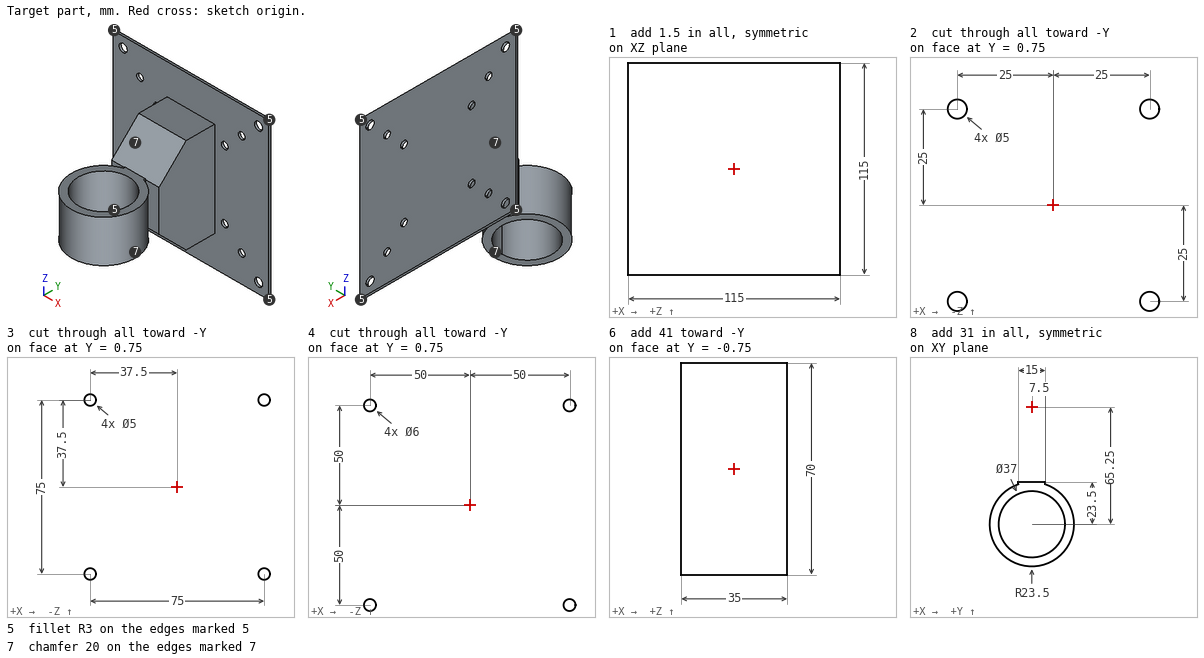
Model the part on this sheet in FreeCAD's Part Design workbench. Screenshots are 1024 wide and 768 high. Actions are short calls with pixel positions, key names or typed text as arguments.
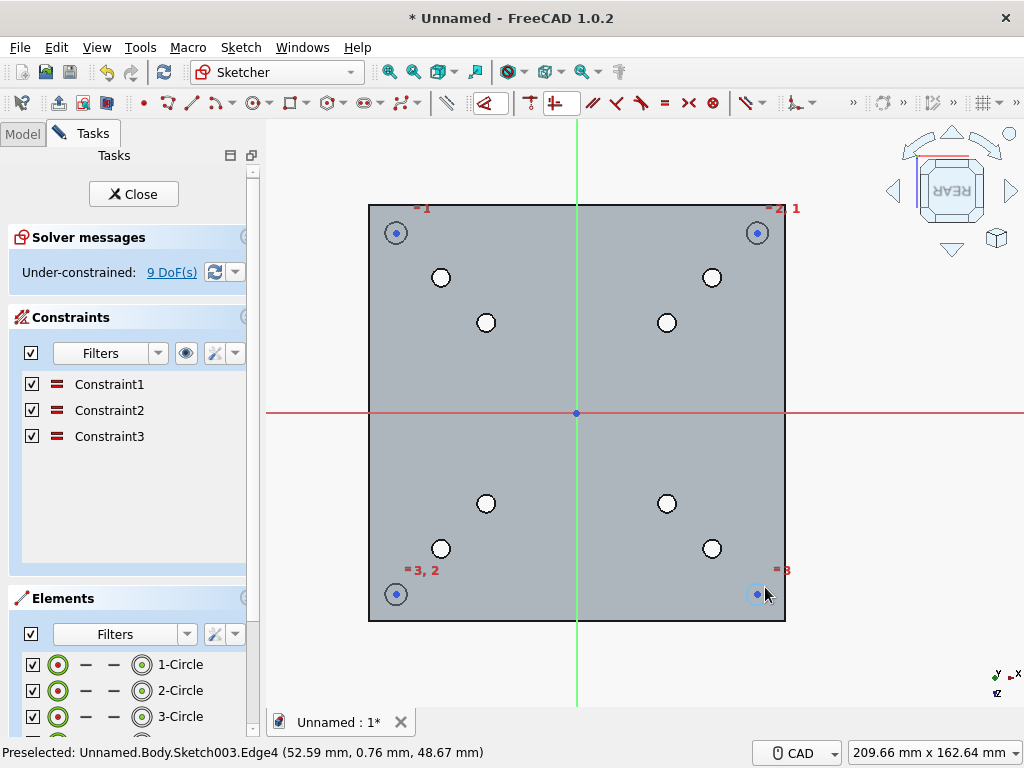
click(396, 233)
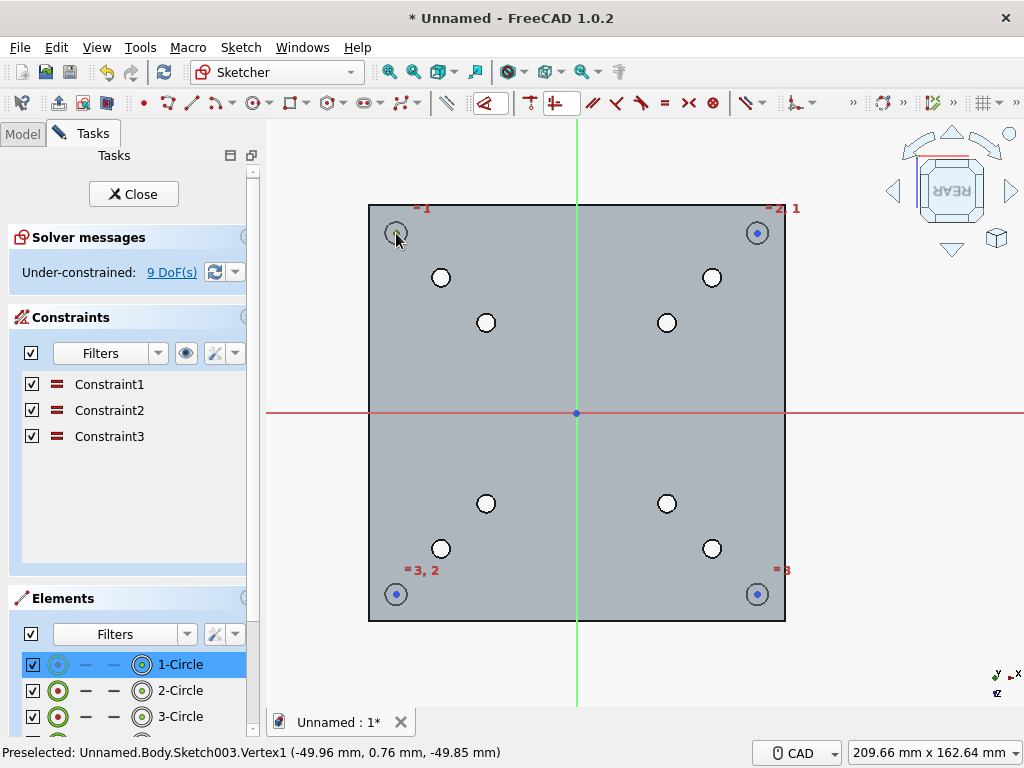
click(757, 233)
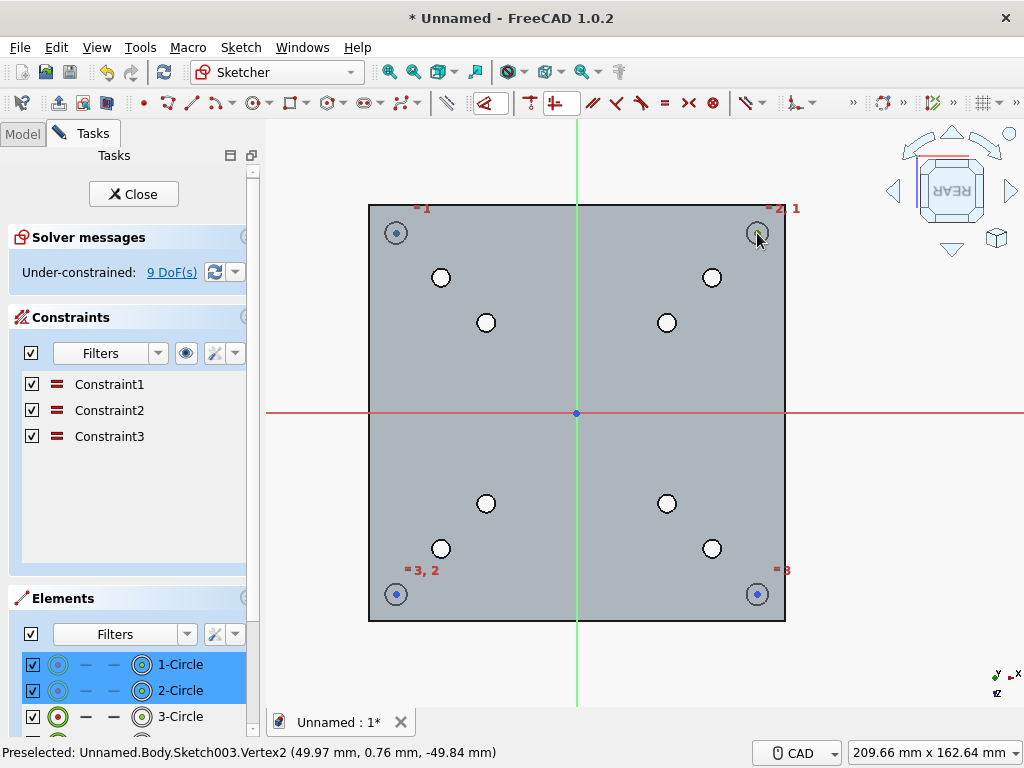
click(574, 104)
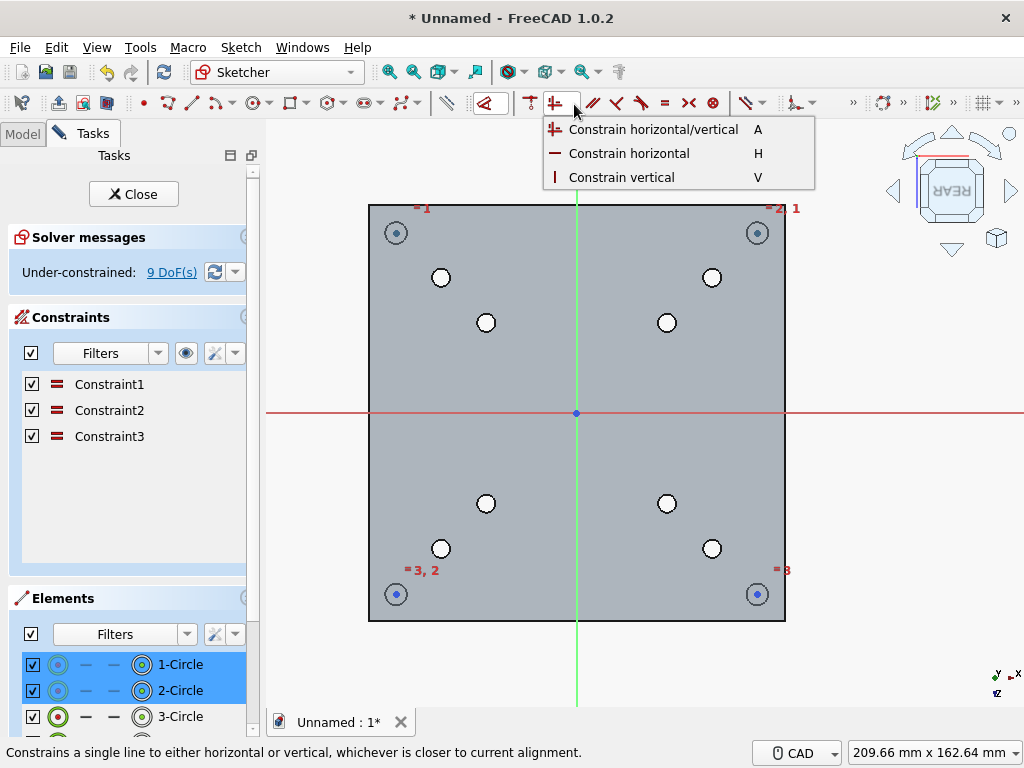
click(679, 153)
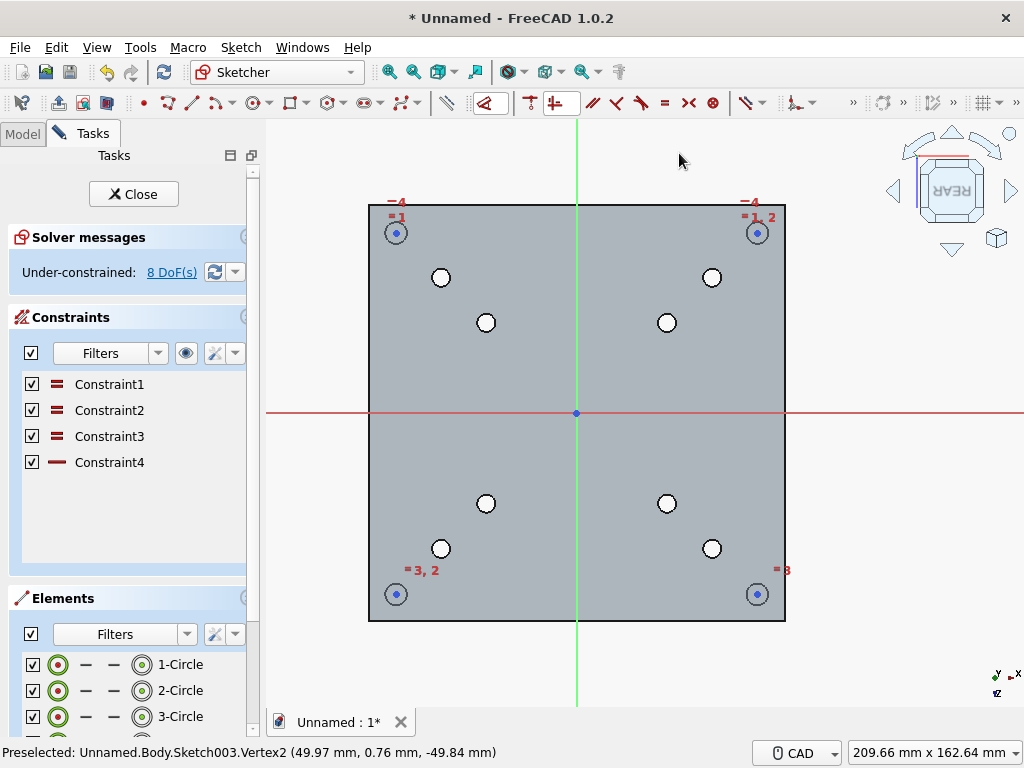
click(396, 233)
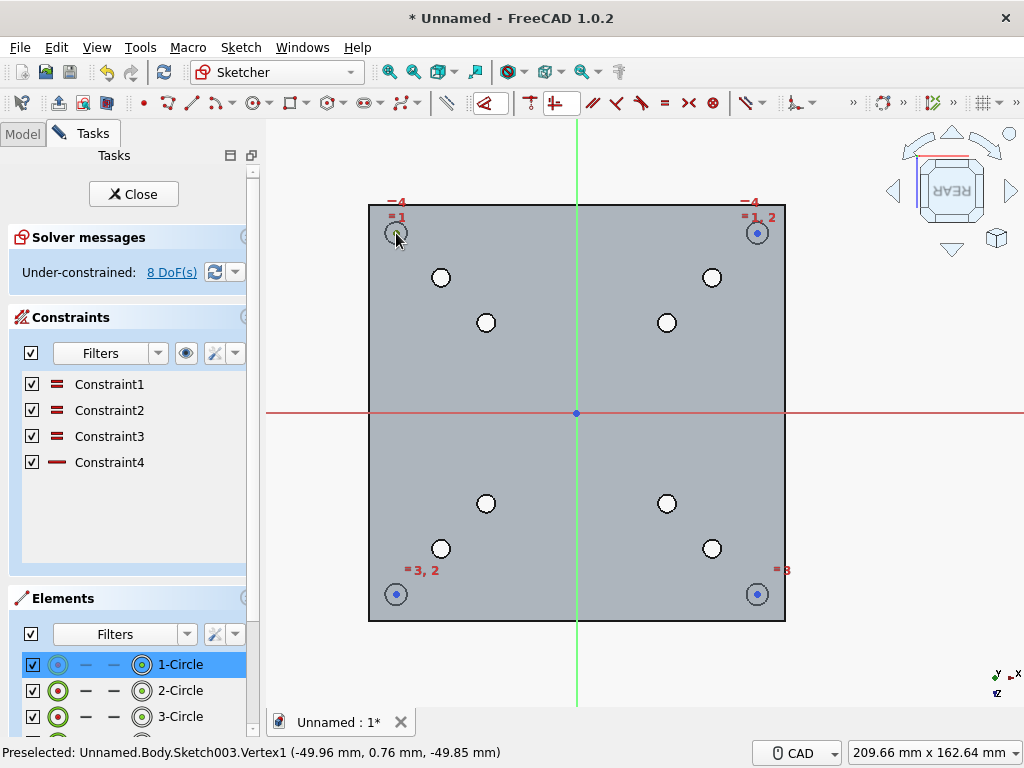
click(396, 594)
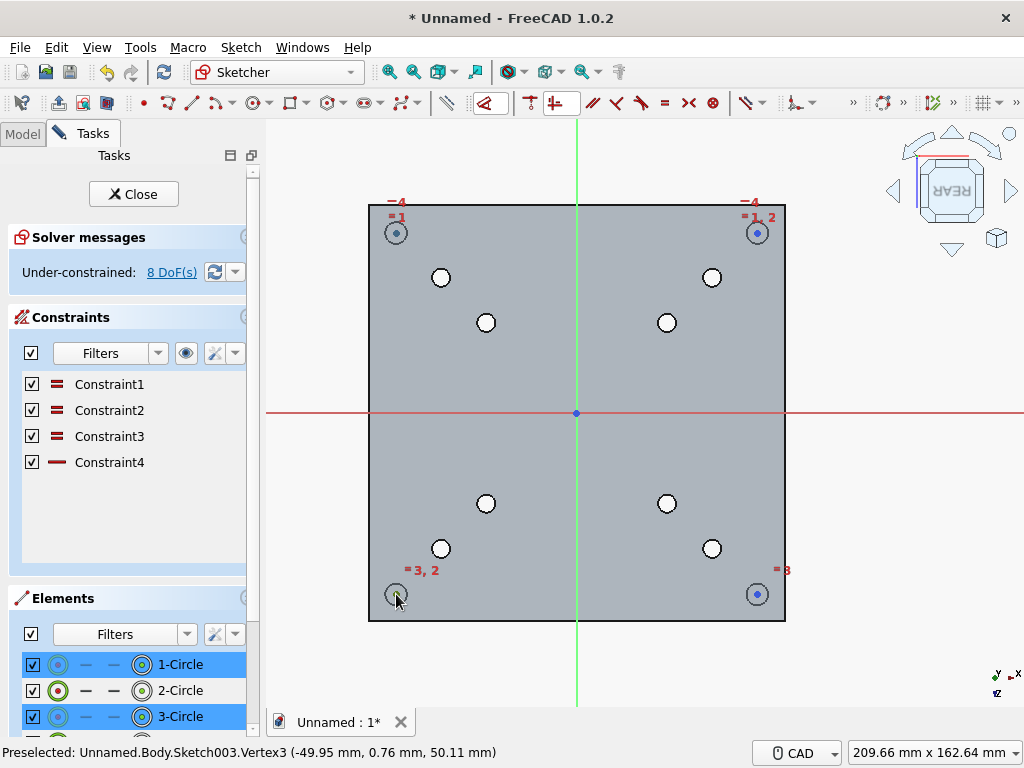
key(v)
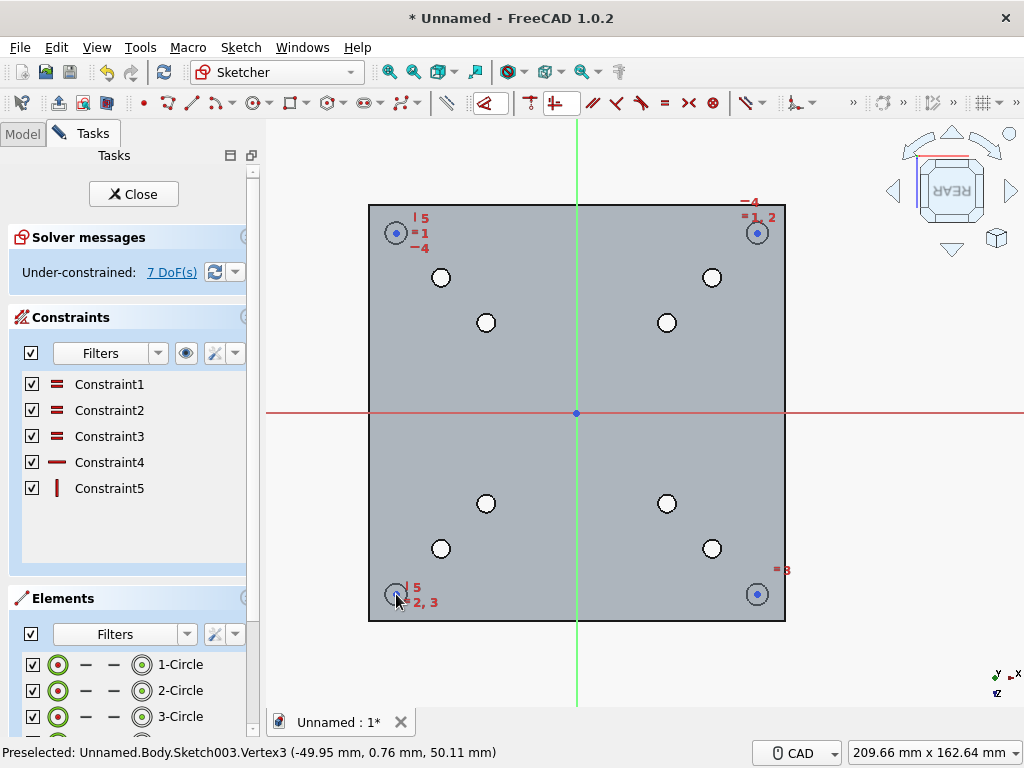
click(757, 233)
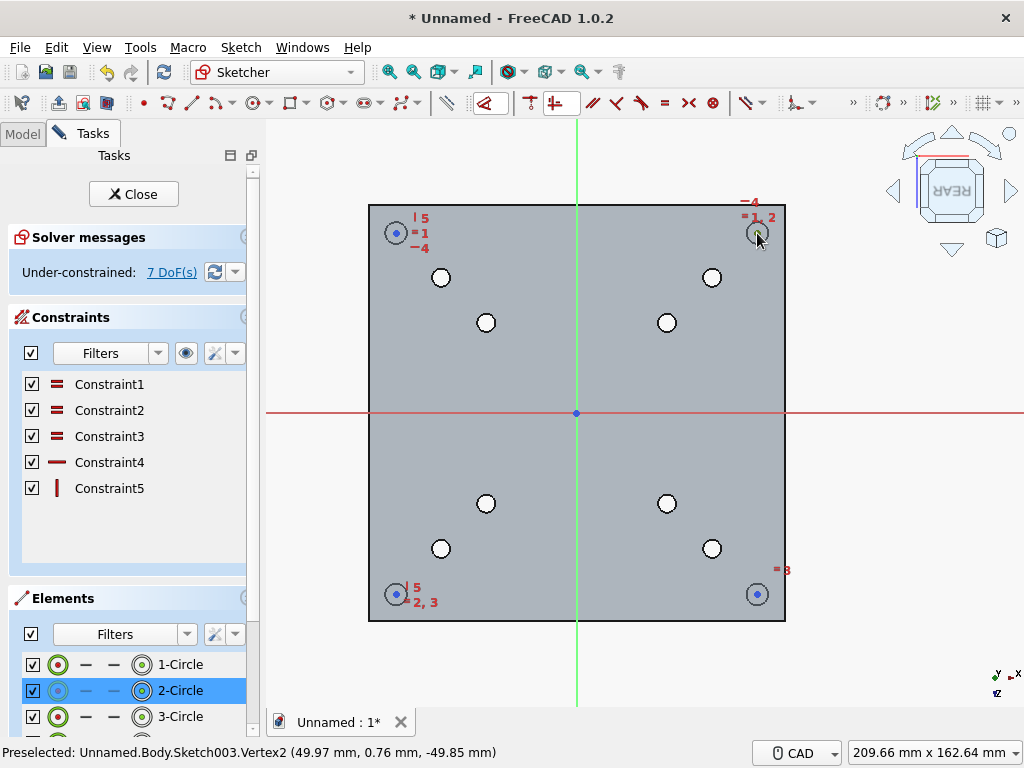
click(757, 594)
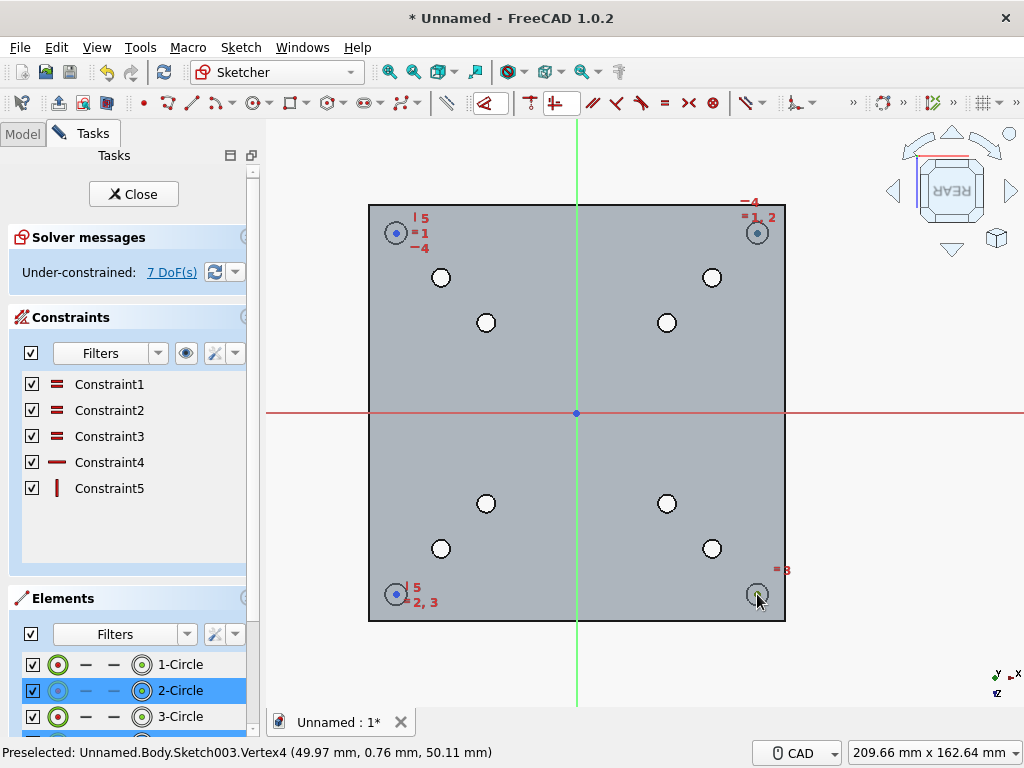
key(v)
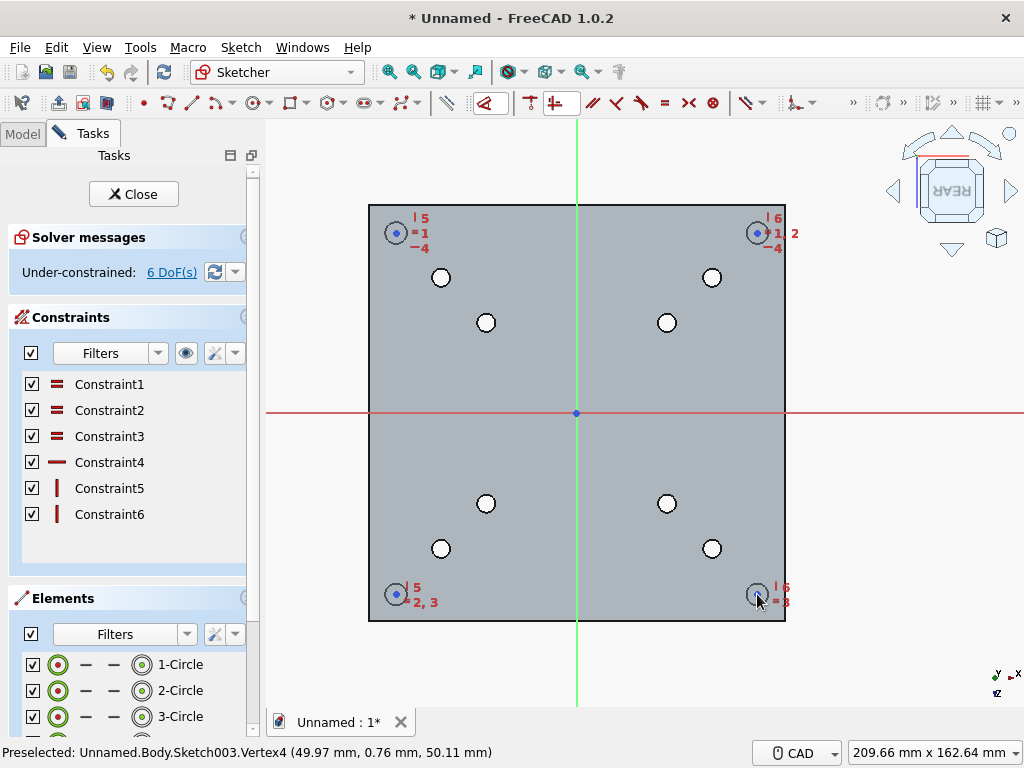
click(396, 594)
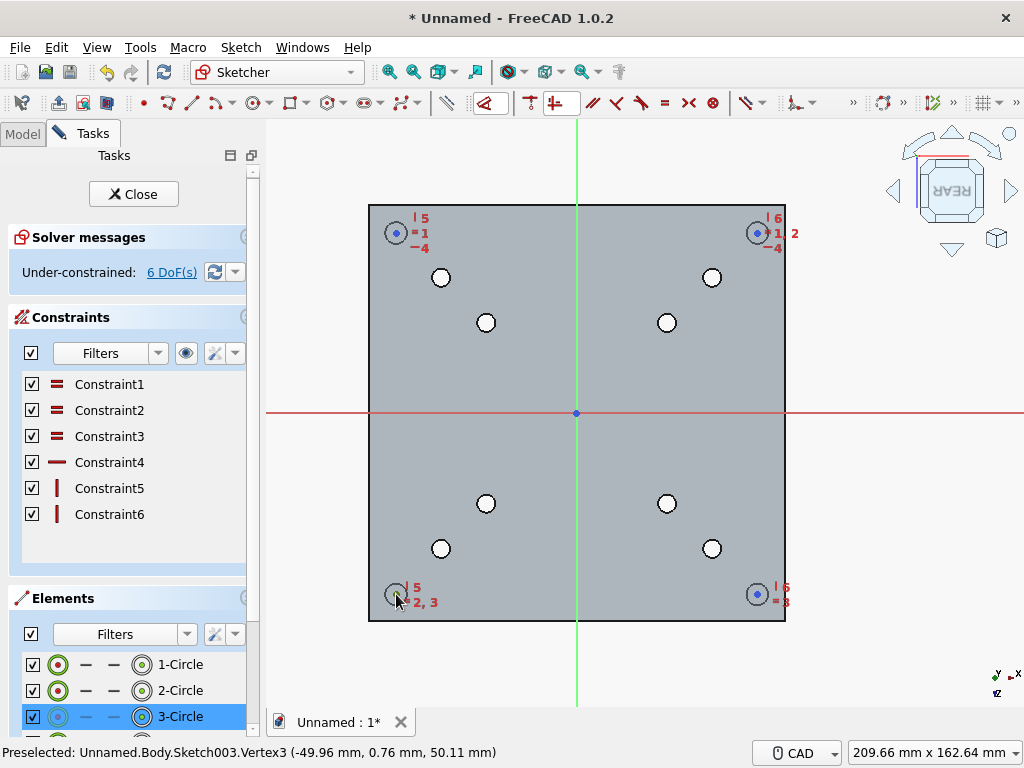
click(757, 594)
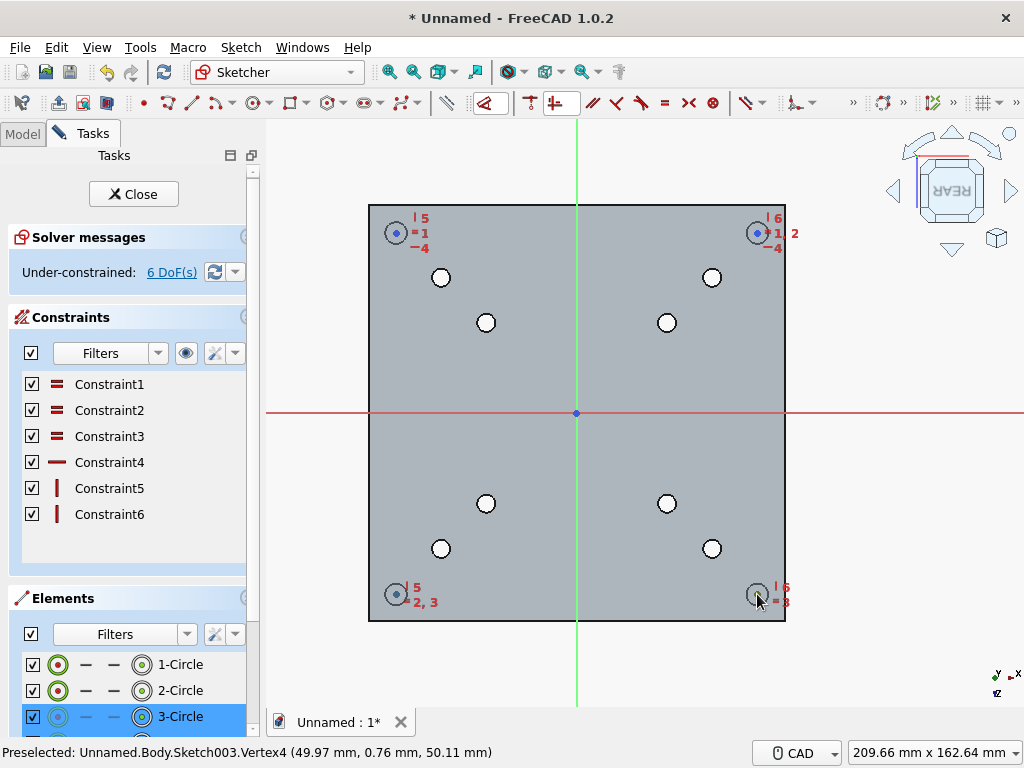
key(h)